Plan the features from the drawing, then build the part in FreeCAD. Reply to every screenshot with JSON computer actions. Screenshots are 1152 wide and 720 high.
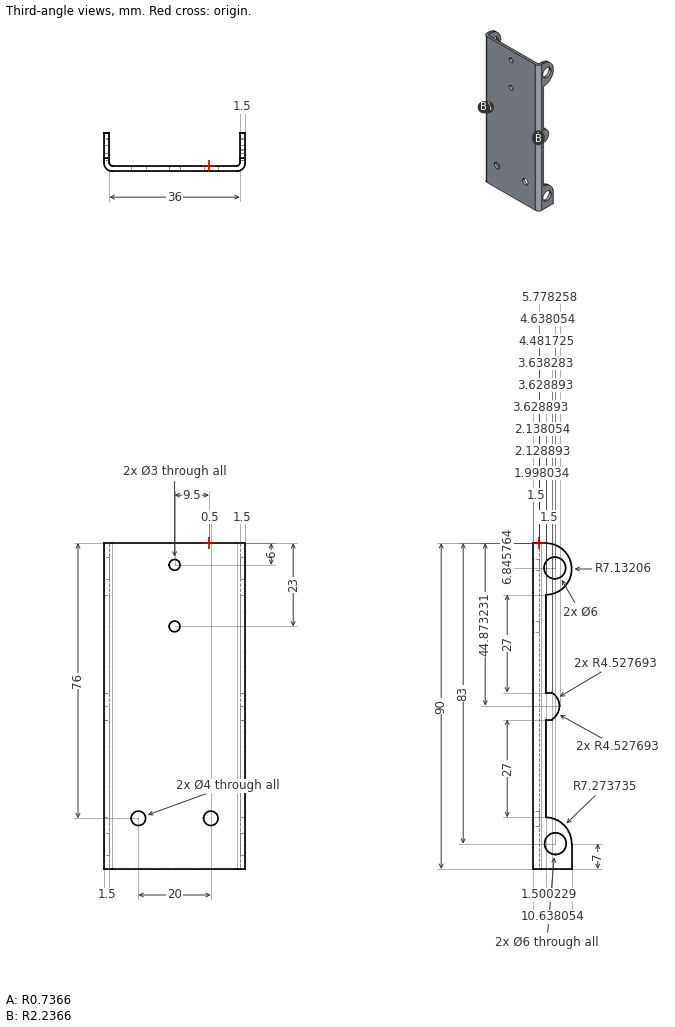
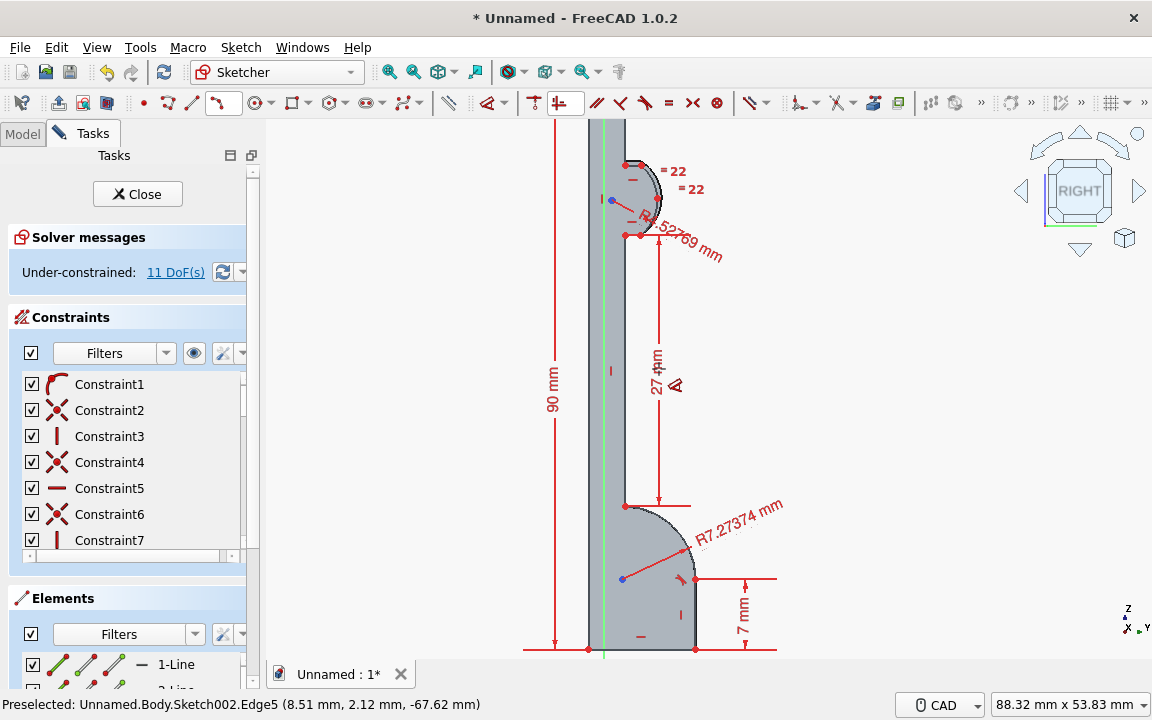
{"action": "scroll", "coordinate": [640, 500], "scroll_direction": "down", "scroll_amount": 5}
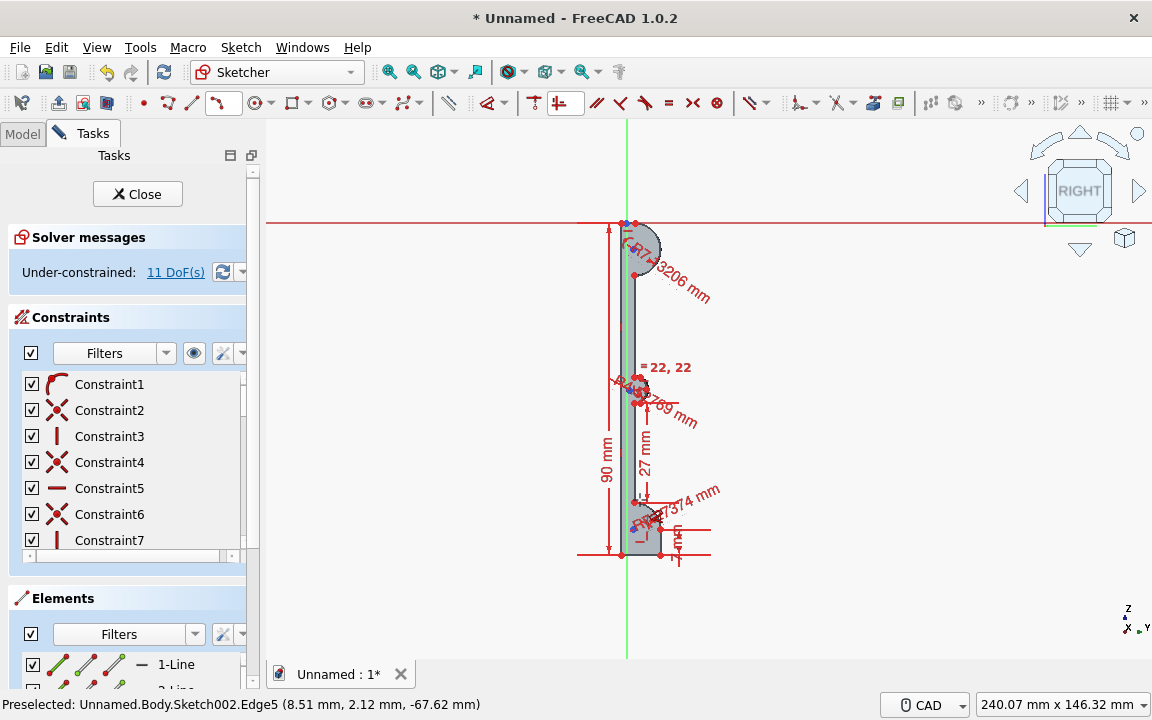
{"action": "scroll", "coordinate": [635, 347], "scroll_direction": "up", "scroll_amount": 3}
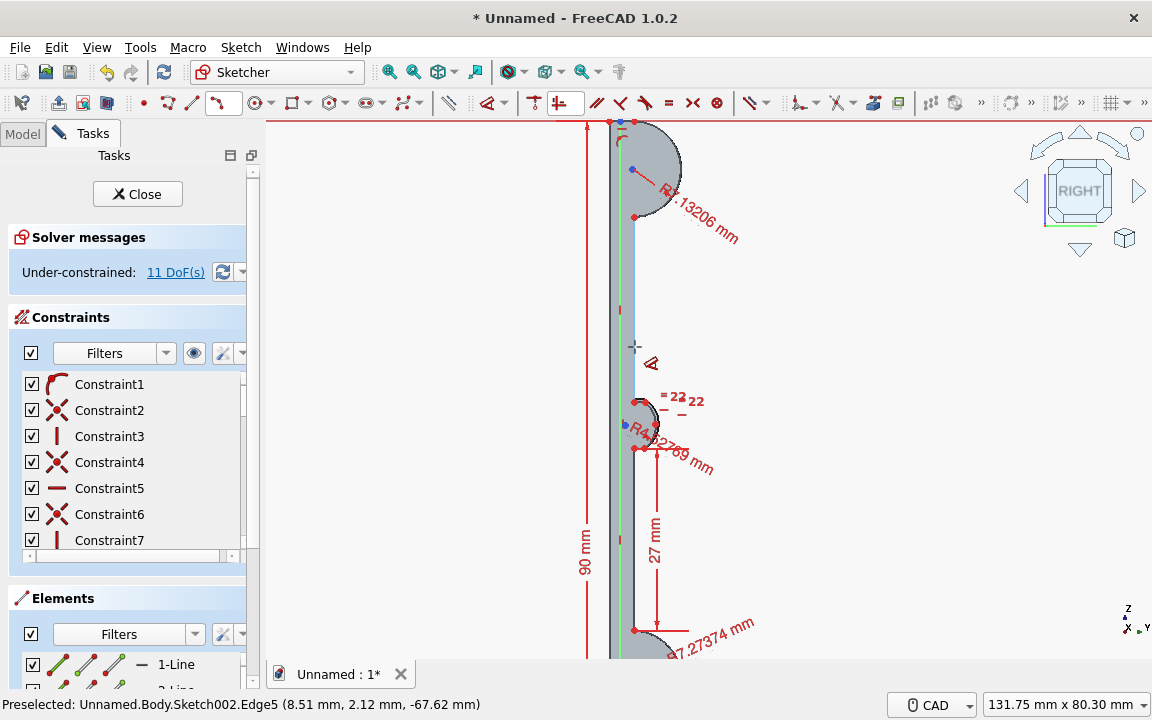
{"action": "left_click", "coordinate": [634, 347]}
{"action": "left_click", "coordinate": [668, 310]}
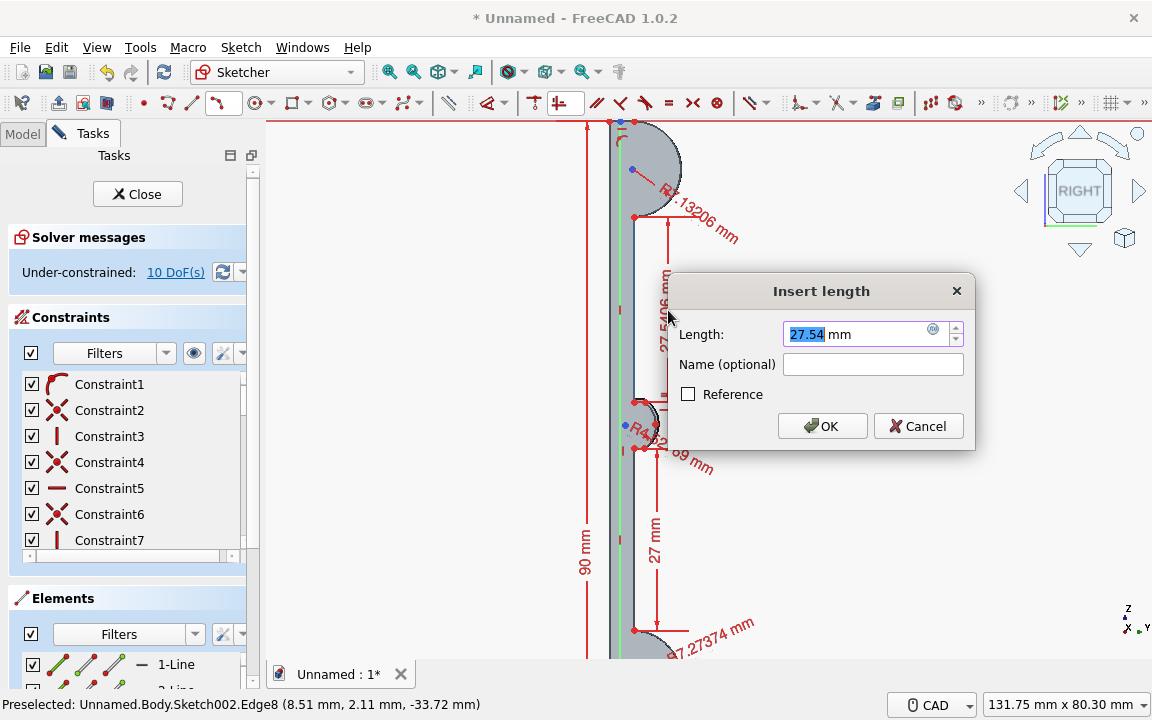
{"action": "type", "text": "27"}
{"action": "key", "text": "Return"}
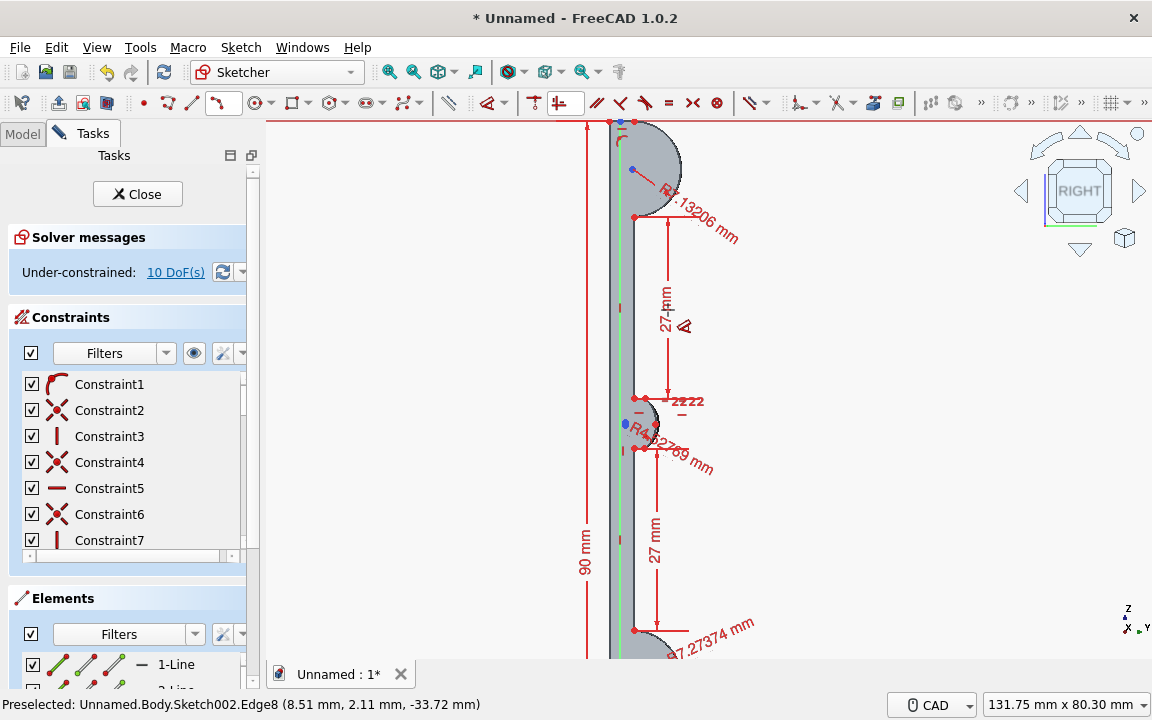
{"action": "scroll", "coordinate": [640, 399], "scroll_direction": "up", "scroll_amount": 7}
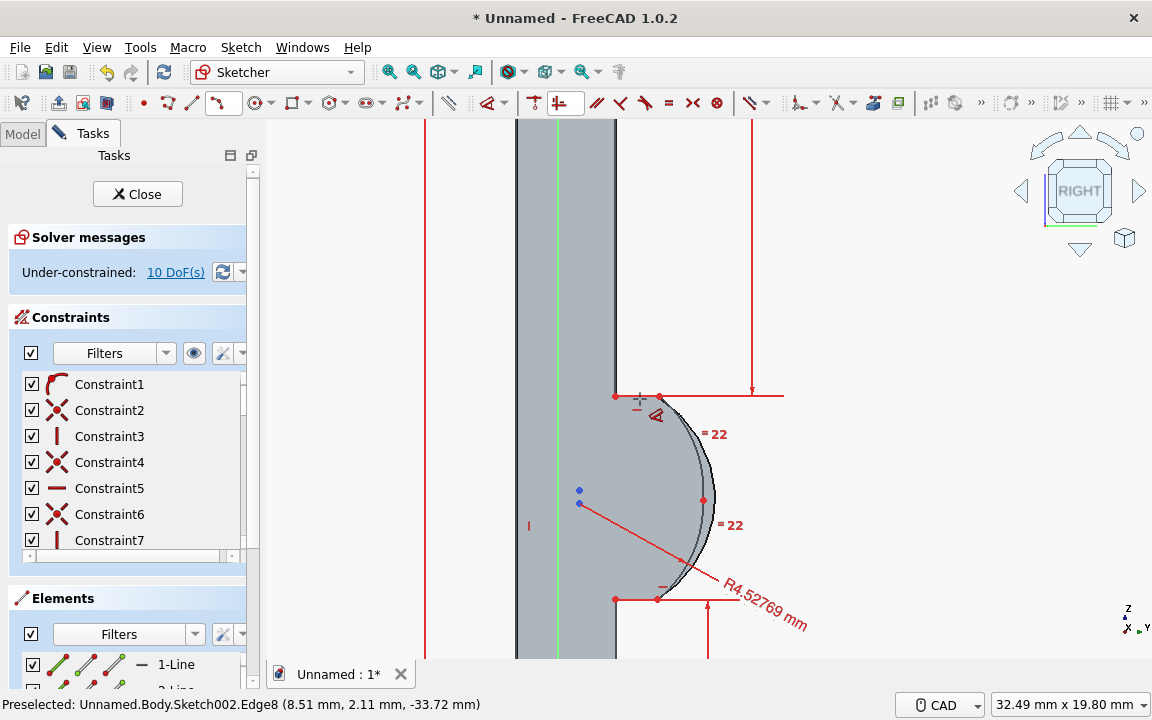
{"action": "left_click", "coordinate": [637, 396]}
{"action": "left_click", "coordinate": [637, 362]}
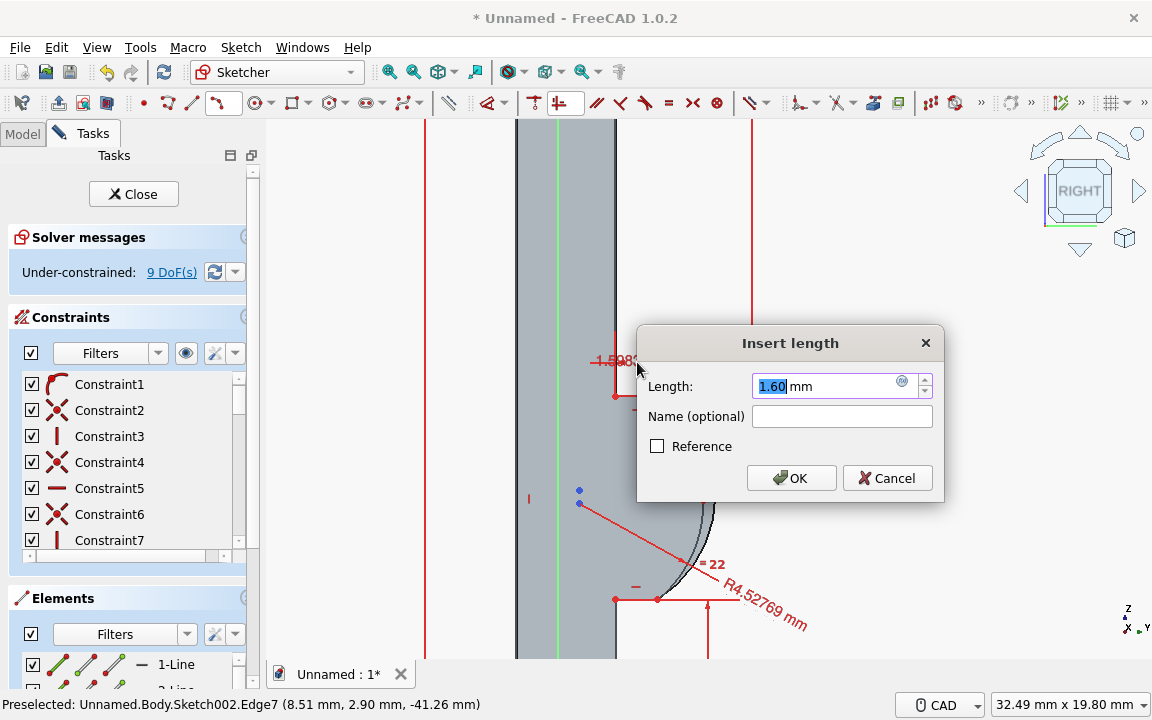
{"action": "type", "text": "1.5"}
{"action": "key", "text": "Return"}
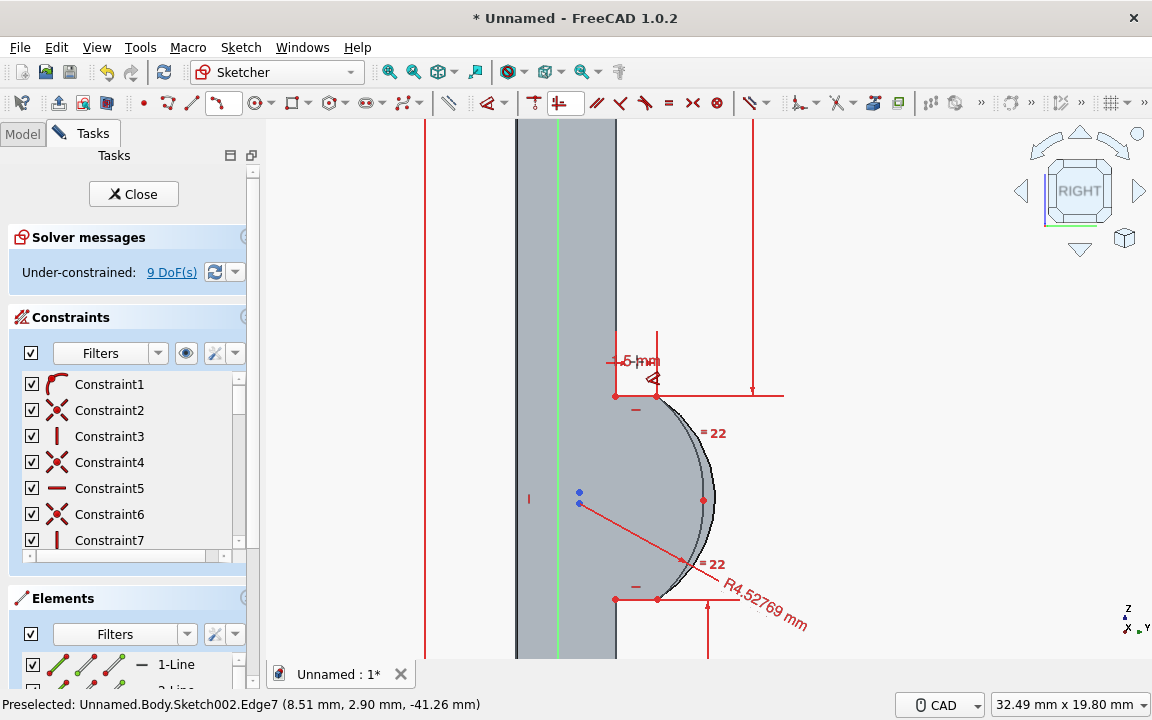
{"action": "scroll", "coordinate": [637, 372], "scroll_direction": "down", "scroll_amount": 10}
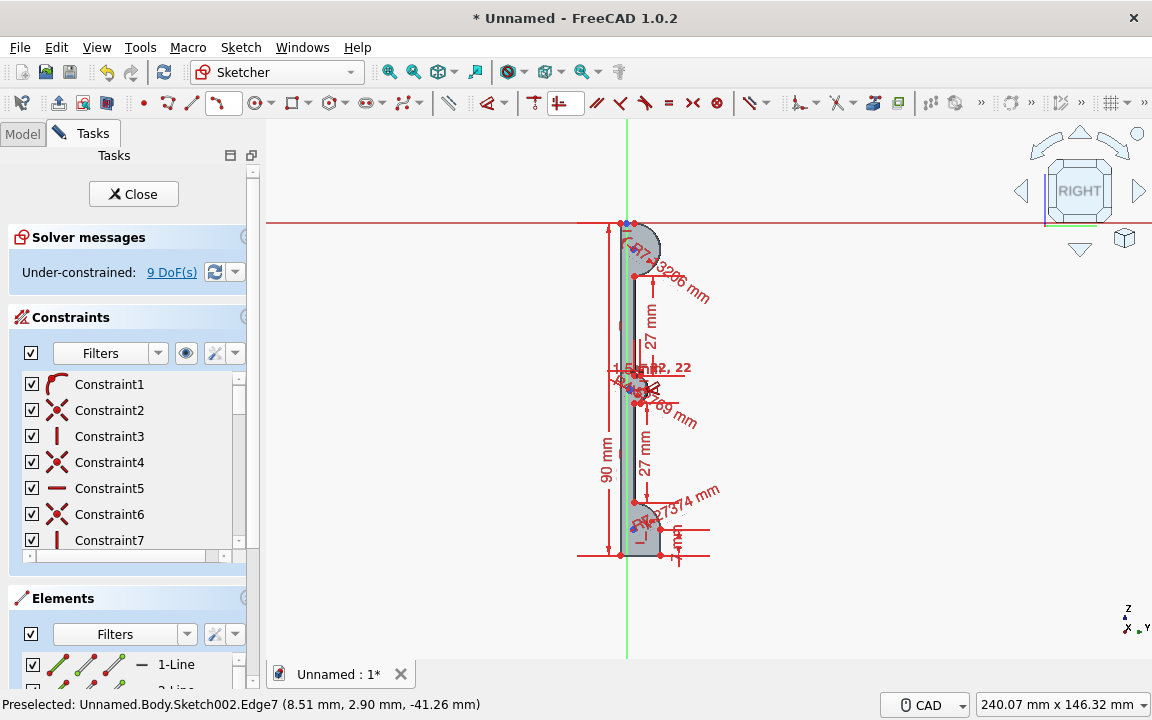
{"action": "scroll", "coordinate": [621, 223], "scroll_direction": "up", "scroll_amount": 10}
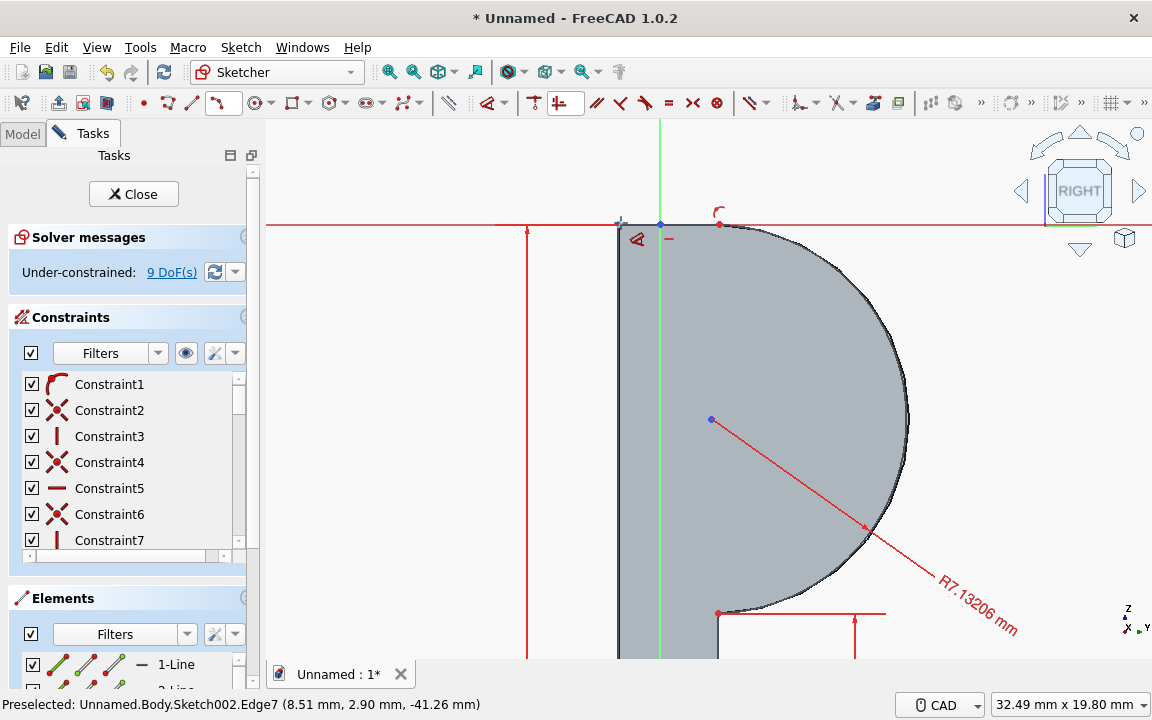
{"action": "left_click", "coordinate": [618, 225]}
{"action": "left_click", "coordinate": [639, 191]}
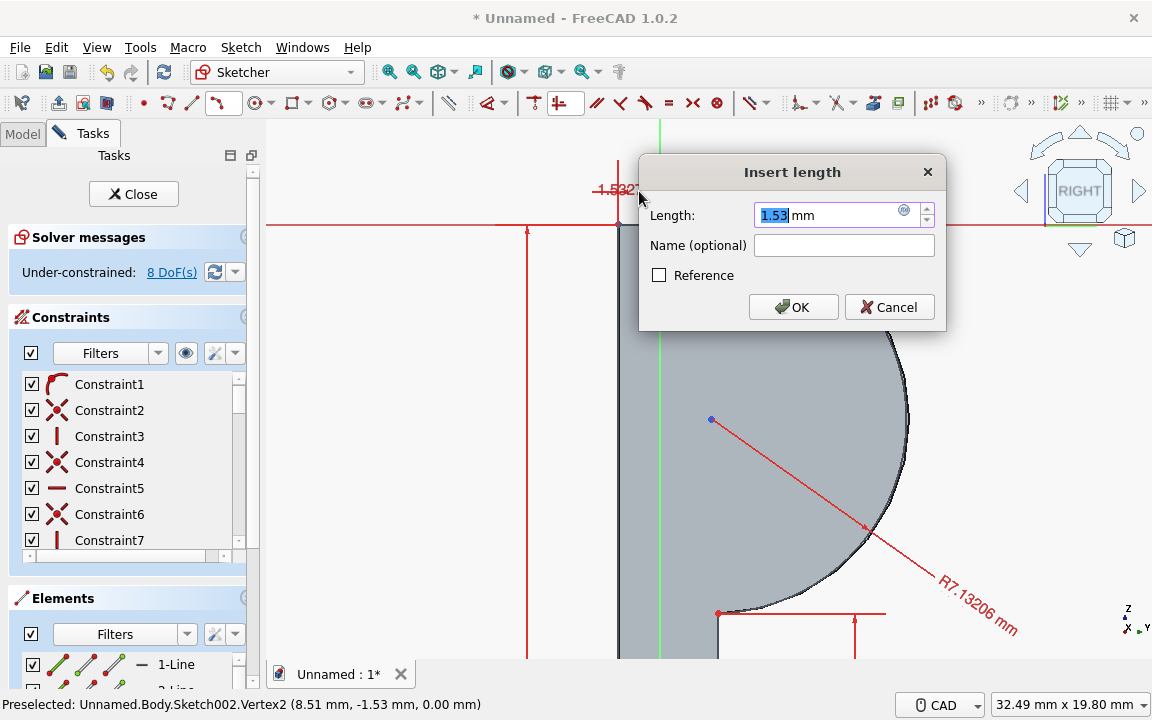
{"action": "type", "text": "1.5"}
{"action": "key", "text": "Return"}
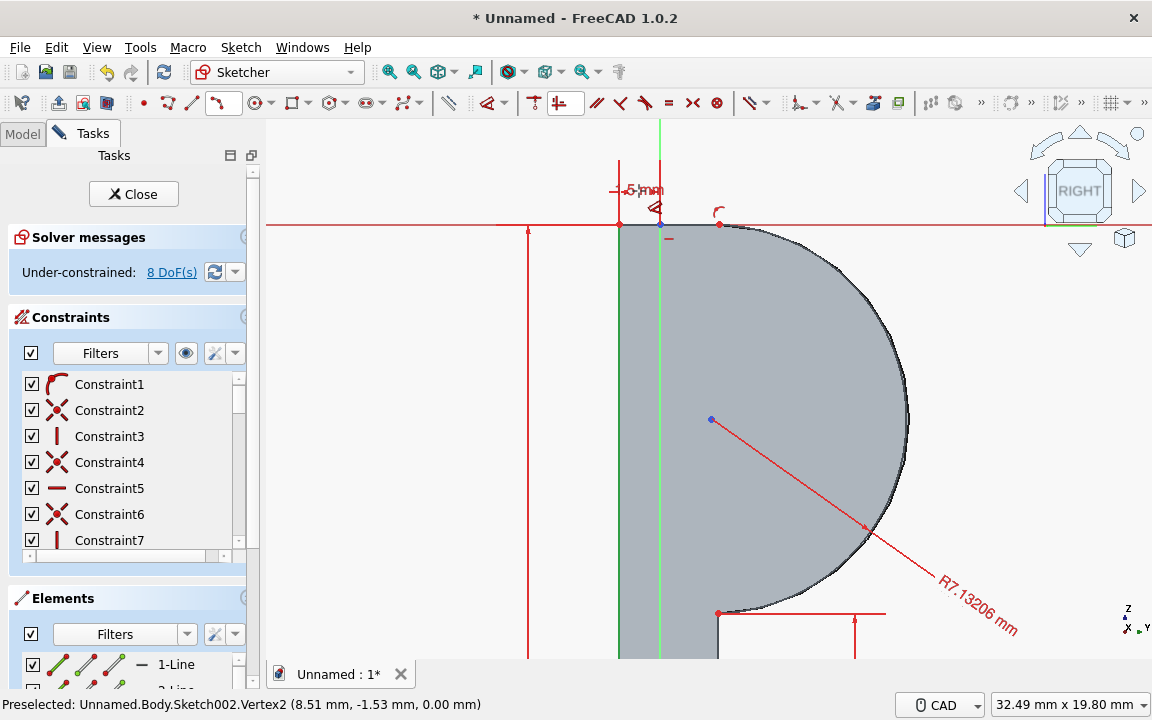
{"action": "left_click", "coordinate": [690, 225]}
{"action": "left_click", "coordinate": [646, 259]}